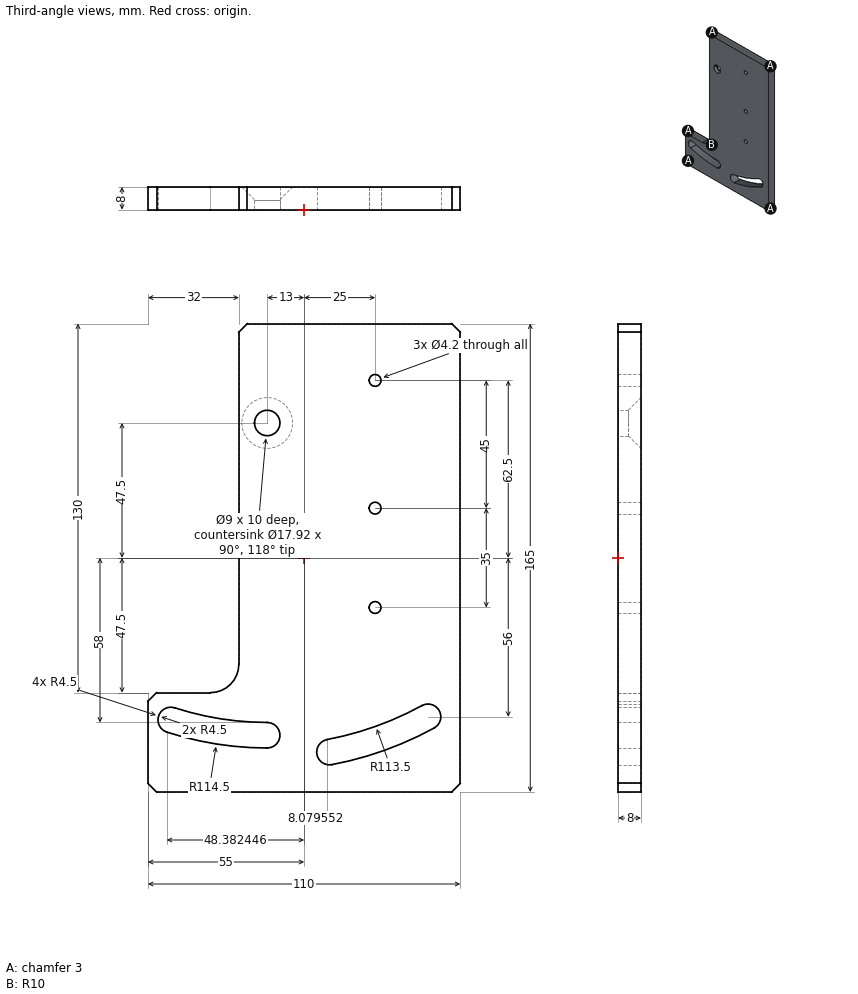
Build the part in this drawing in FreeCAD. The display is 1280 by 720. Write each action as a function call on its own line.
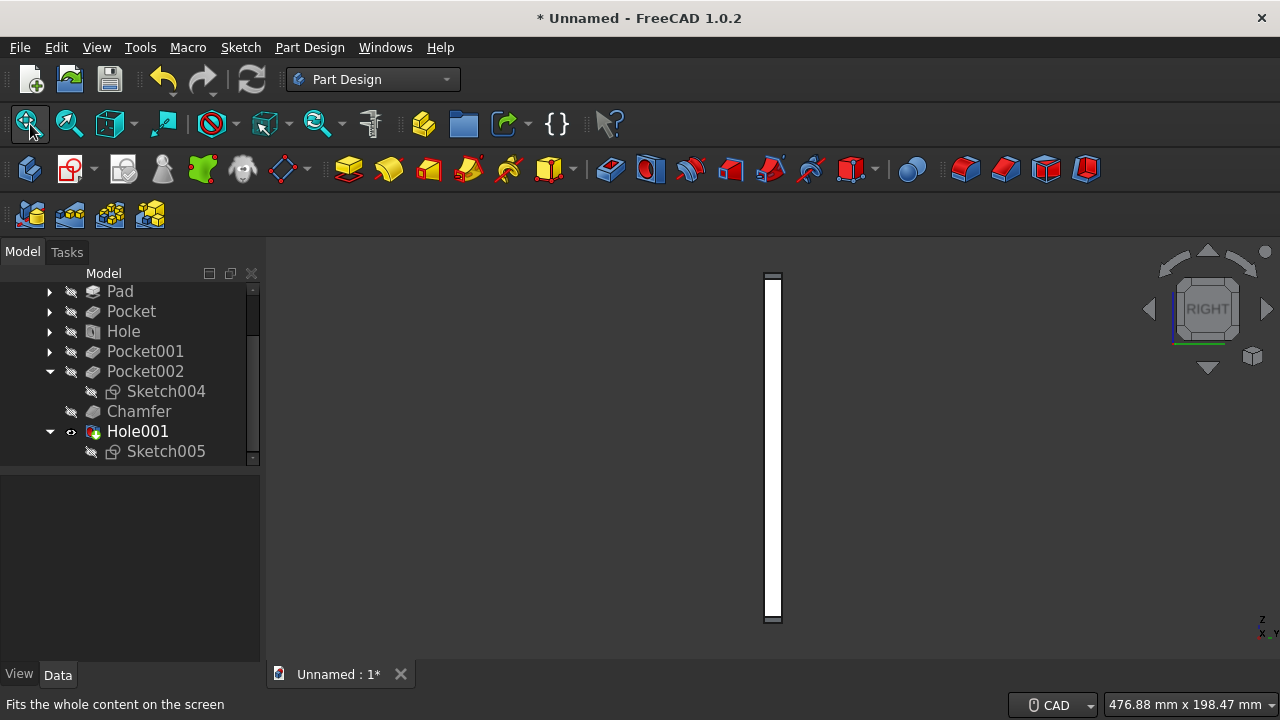
key(5)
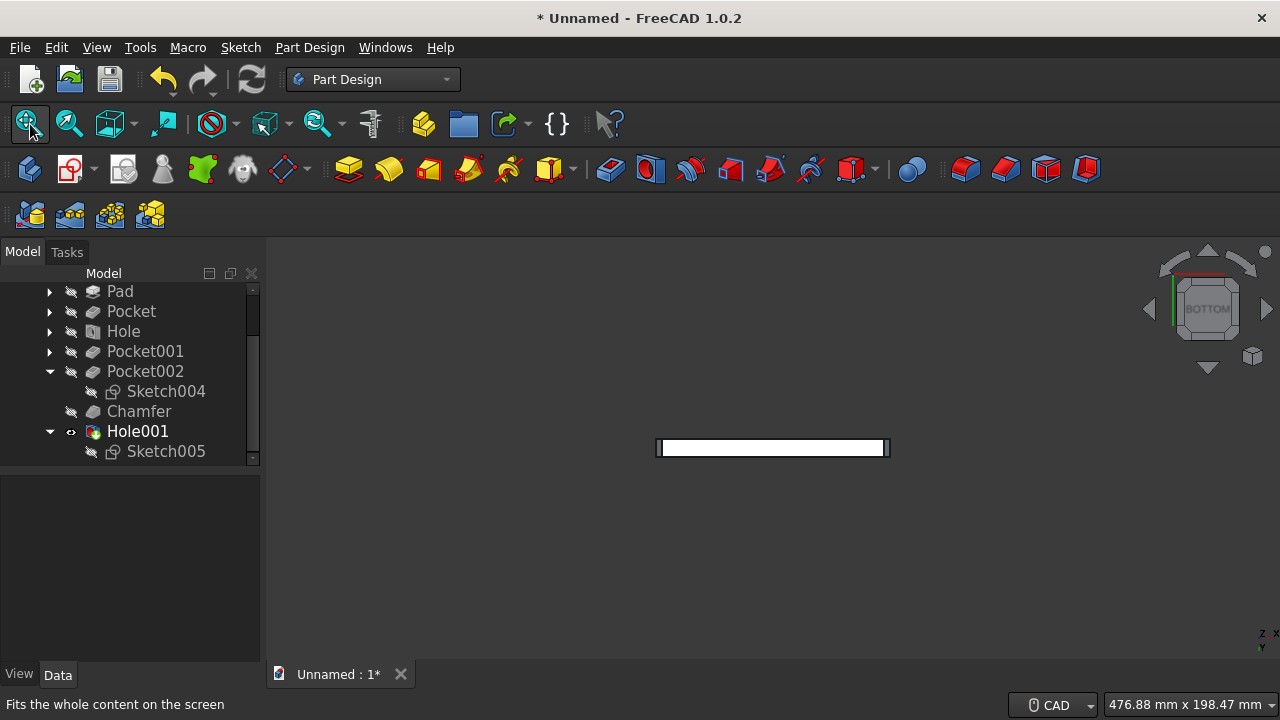
click(30, 124)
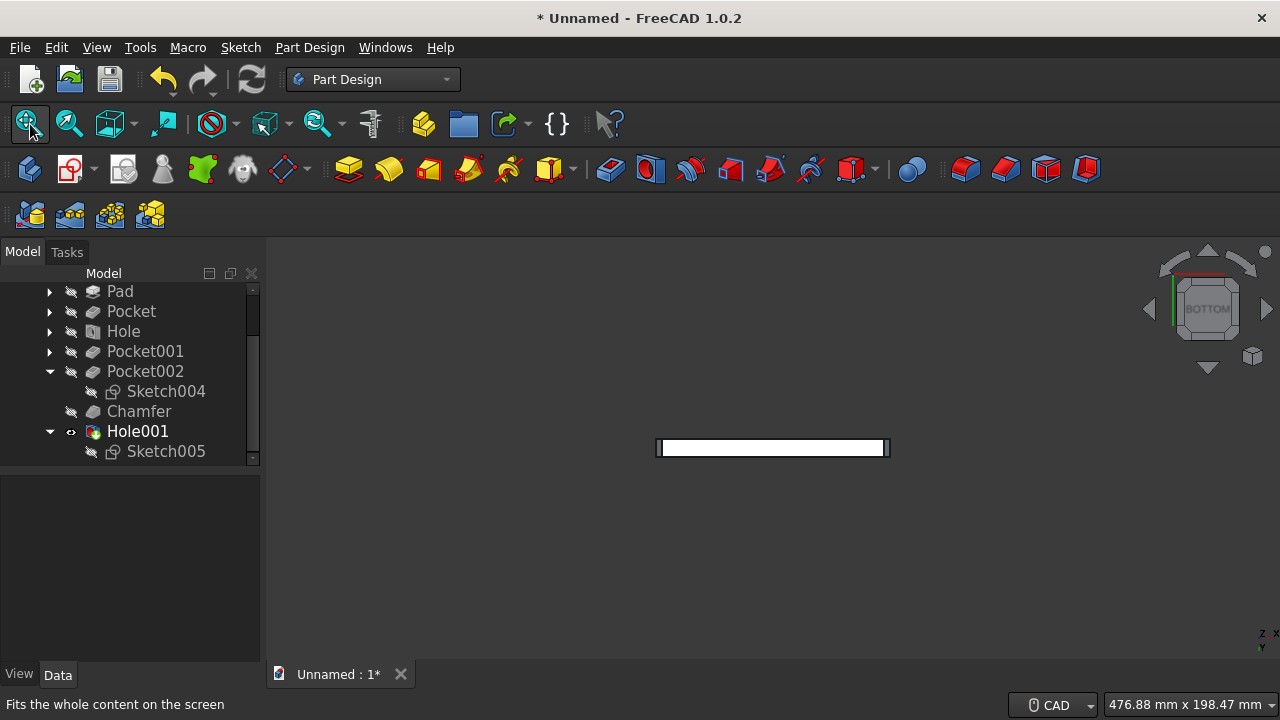
scroll(724, 447, up, 5)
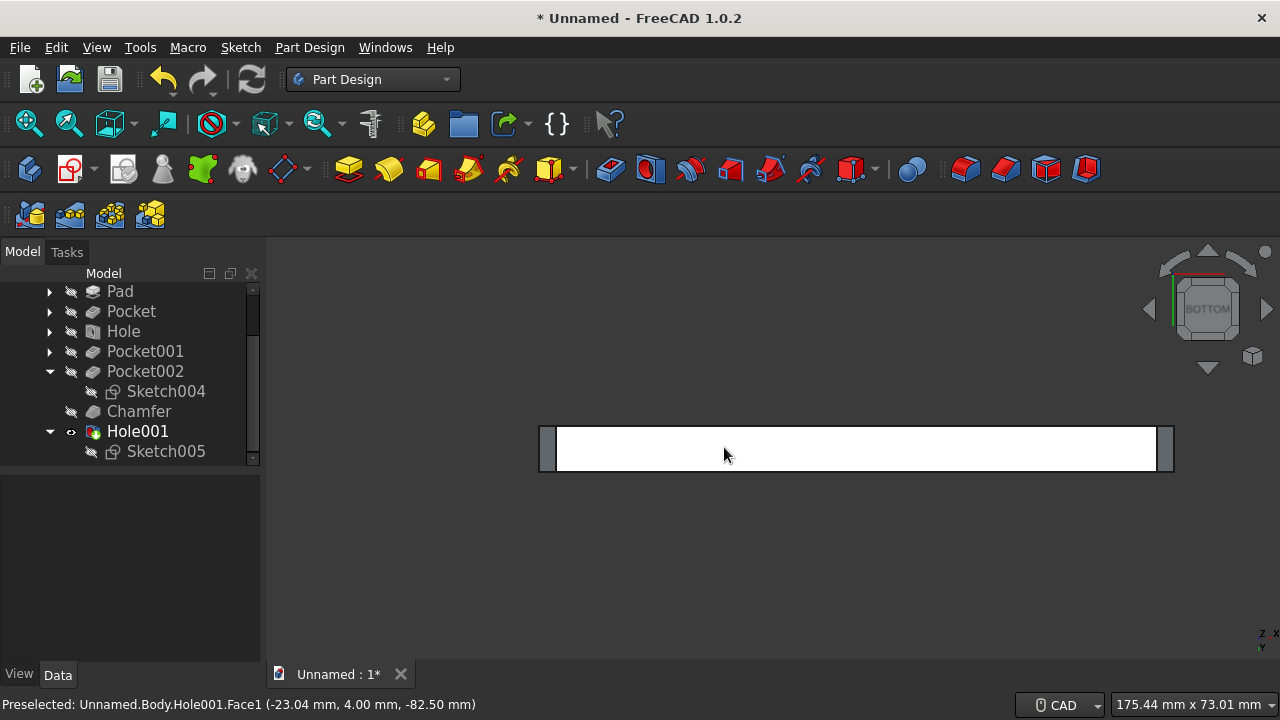
click(30, 124)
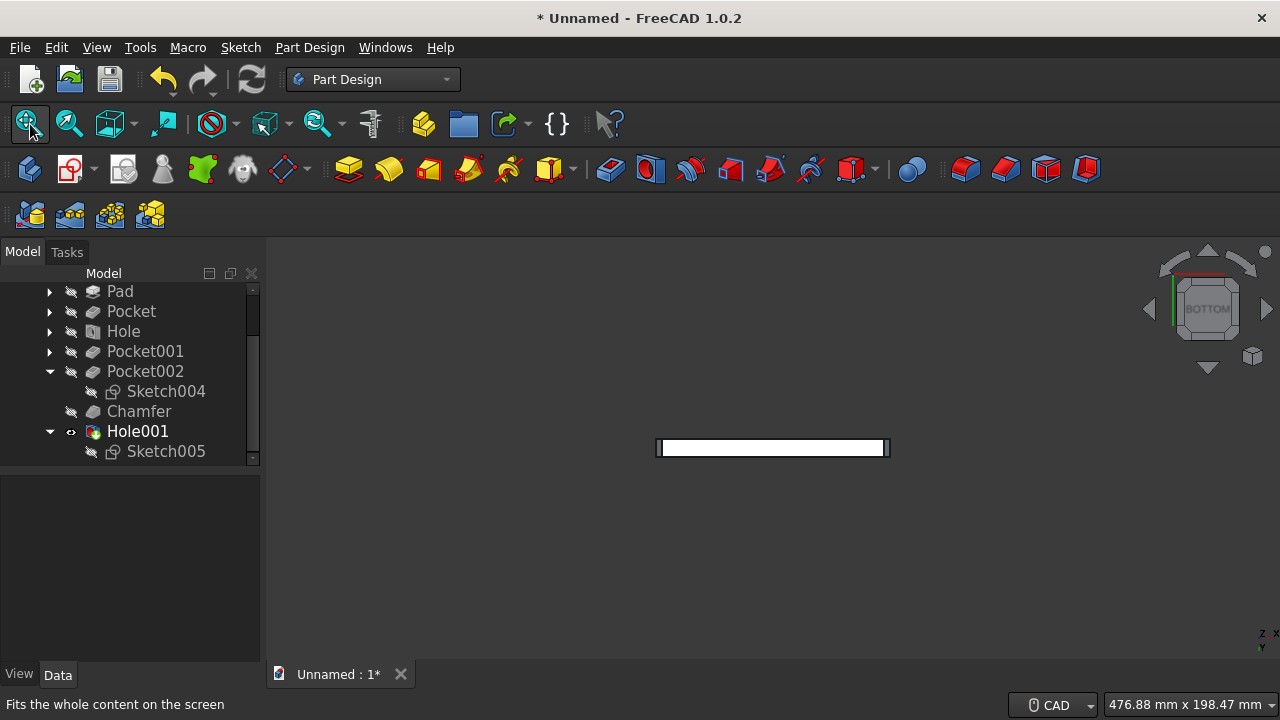
key(4)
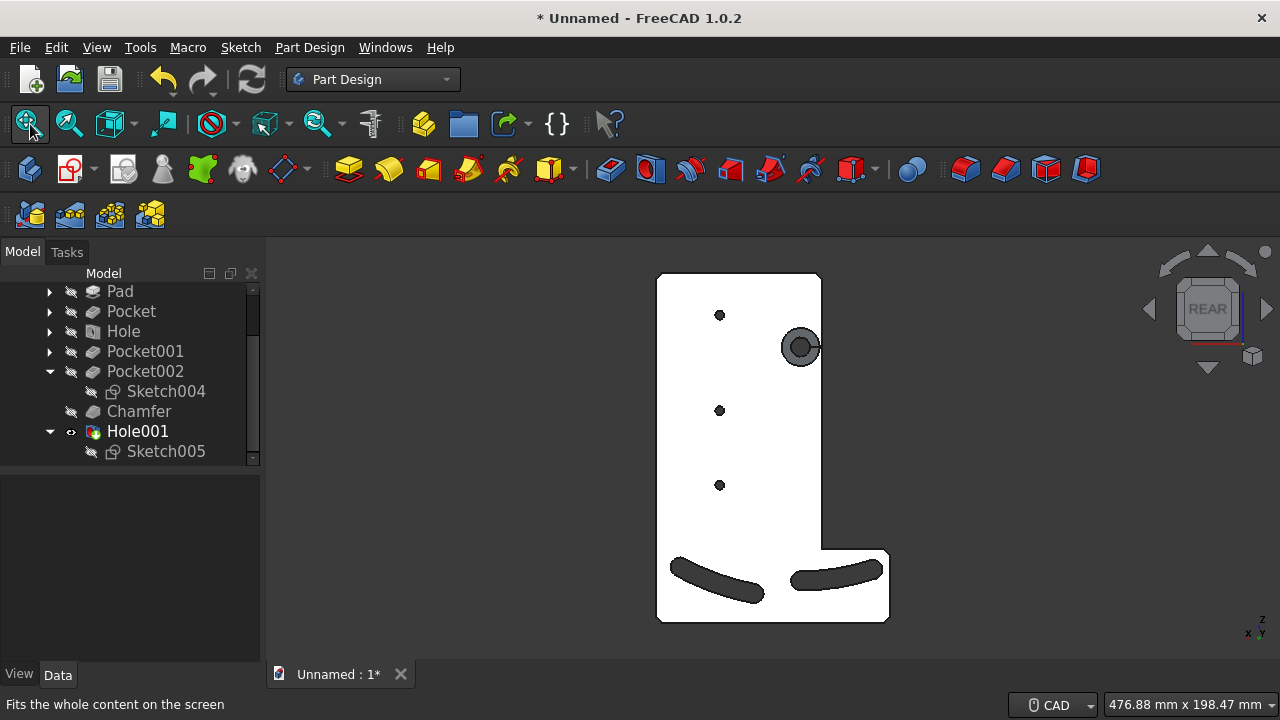
scroll(822, 548, up, 5)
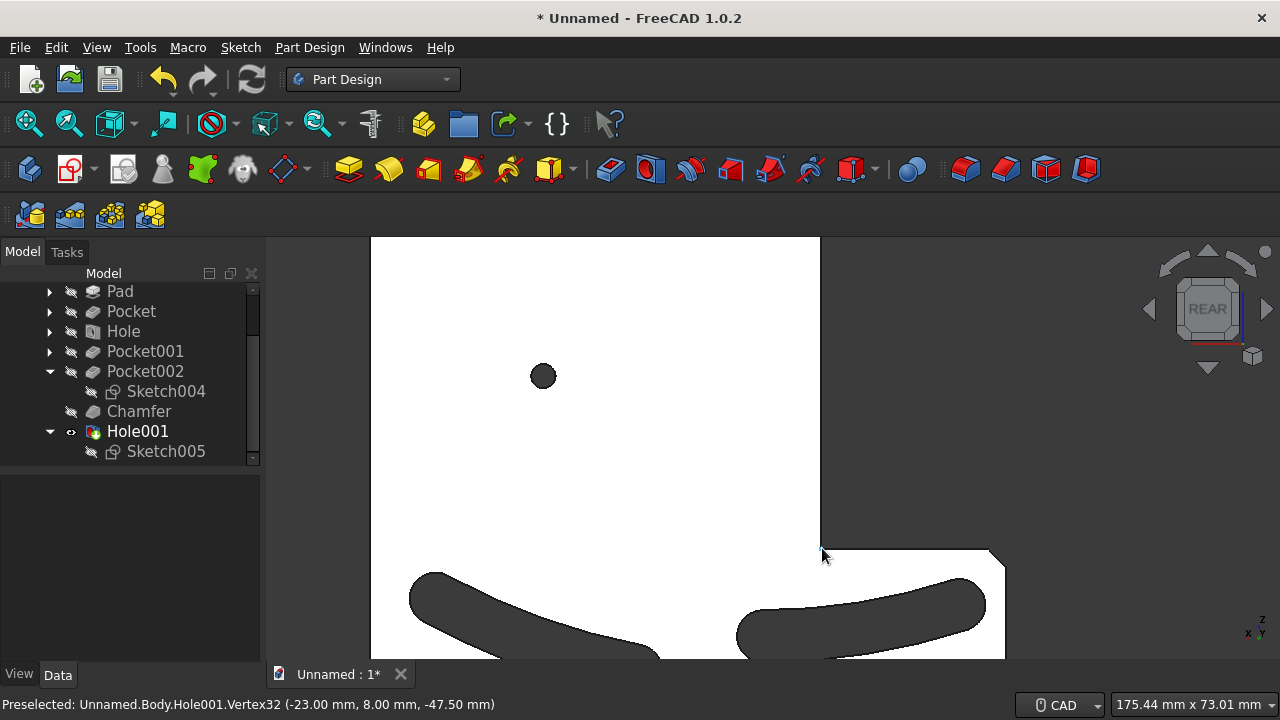
click(30, 124)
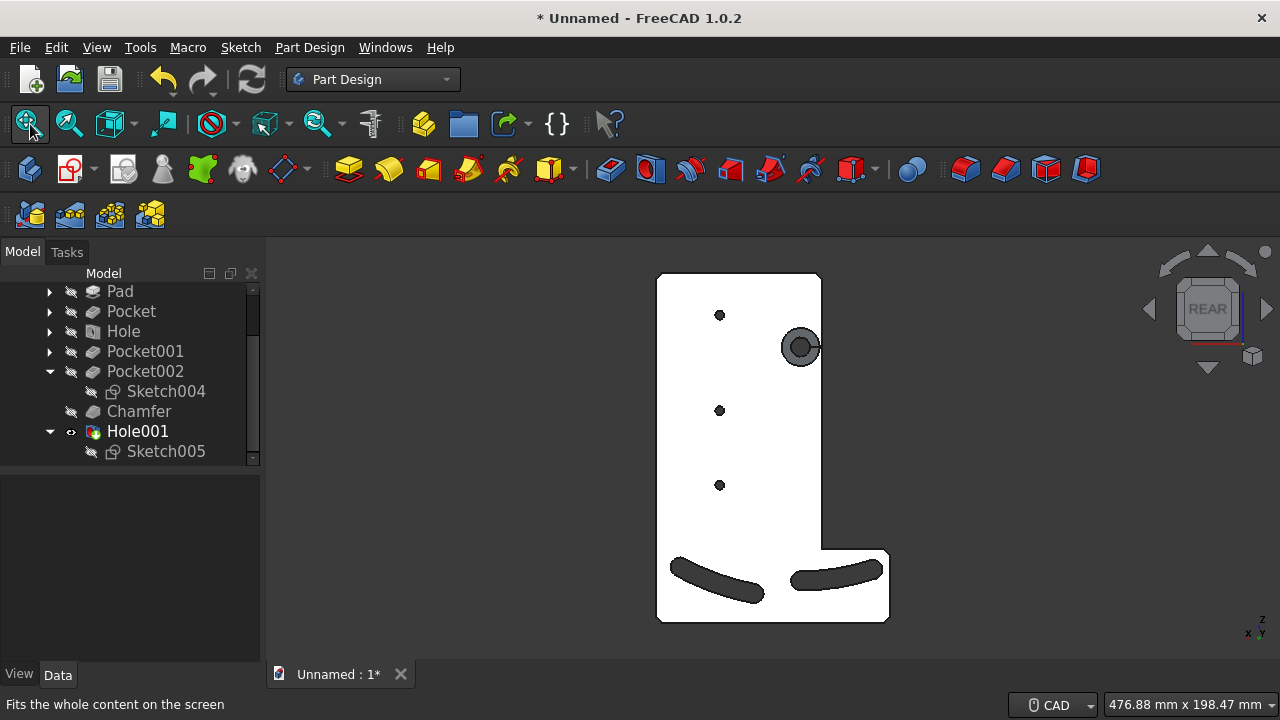
key(6)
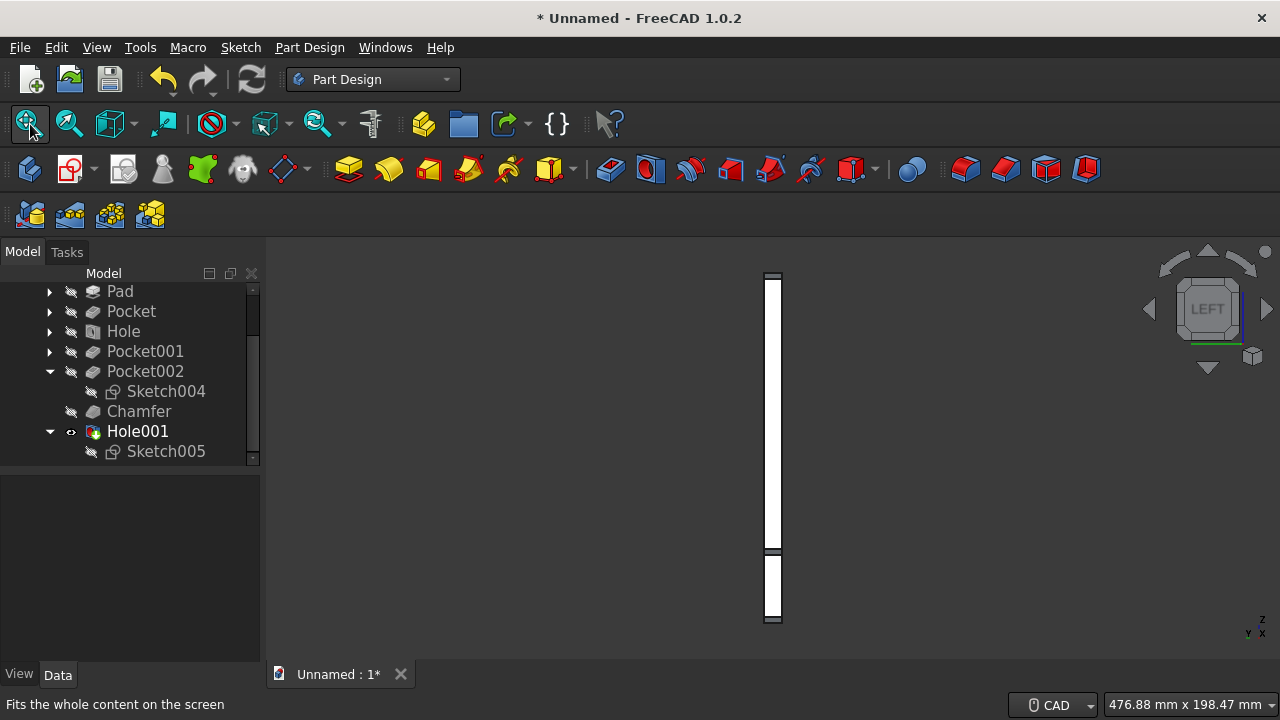
scroll(773, 548, up, 5)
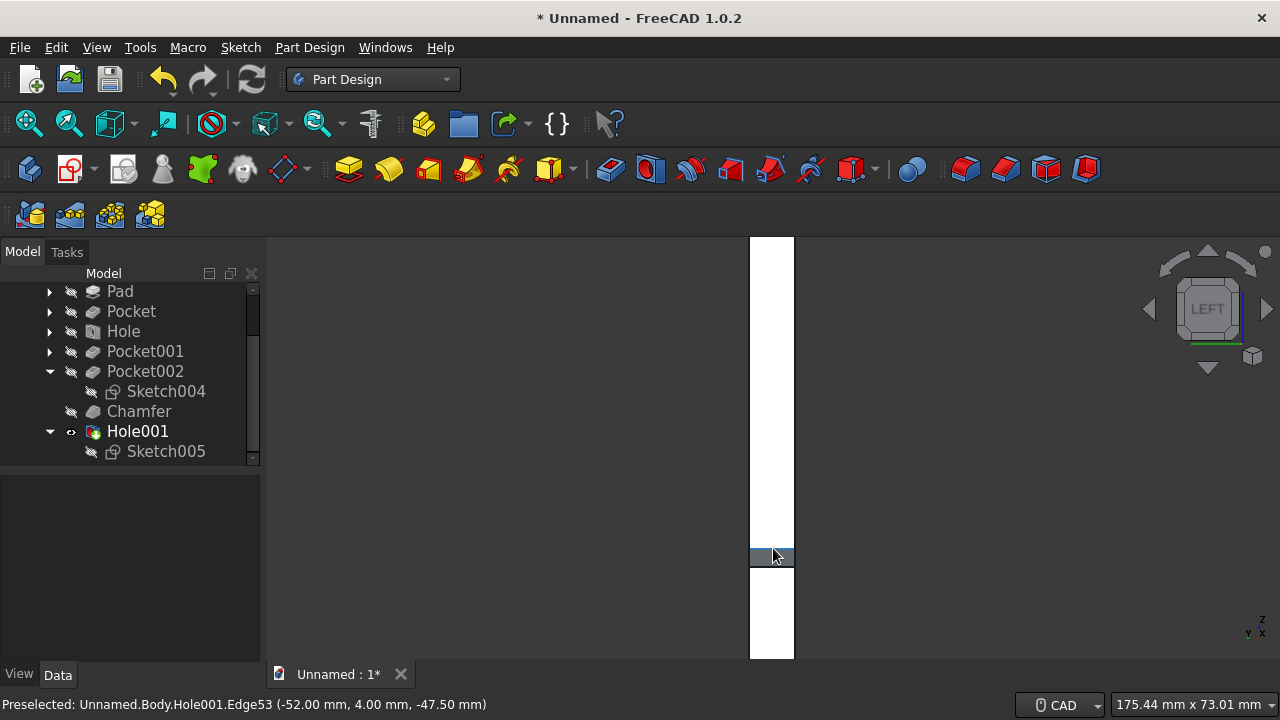
click(30, 124)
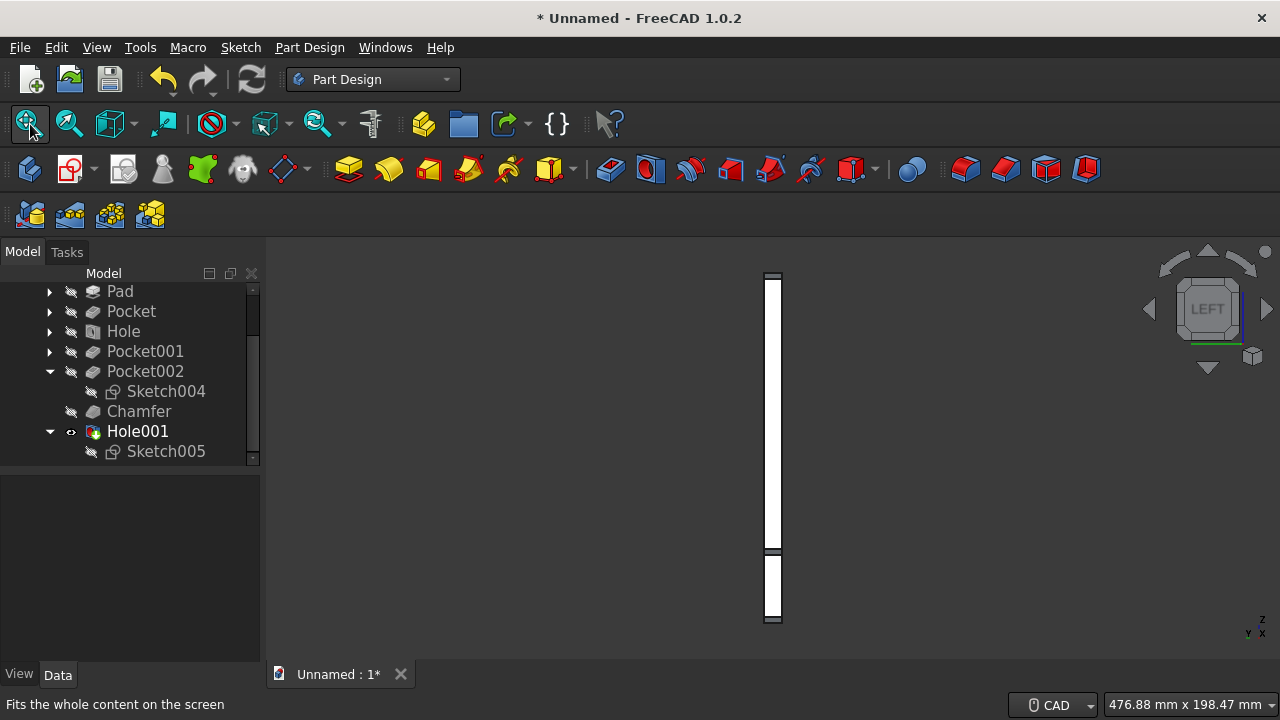
key(v)
key(3)